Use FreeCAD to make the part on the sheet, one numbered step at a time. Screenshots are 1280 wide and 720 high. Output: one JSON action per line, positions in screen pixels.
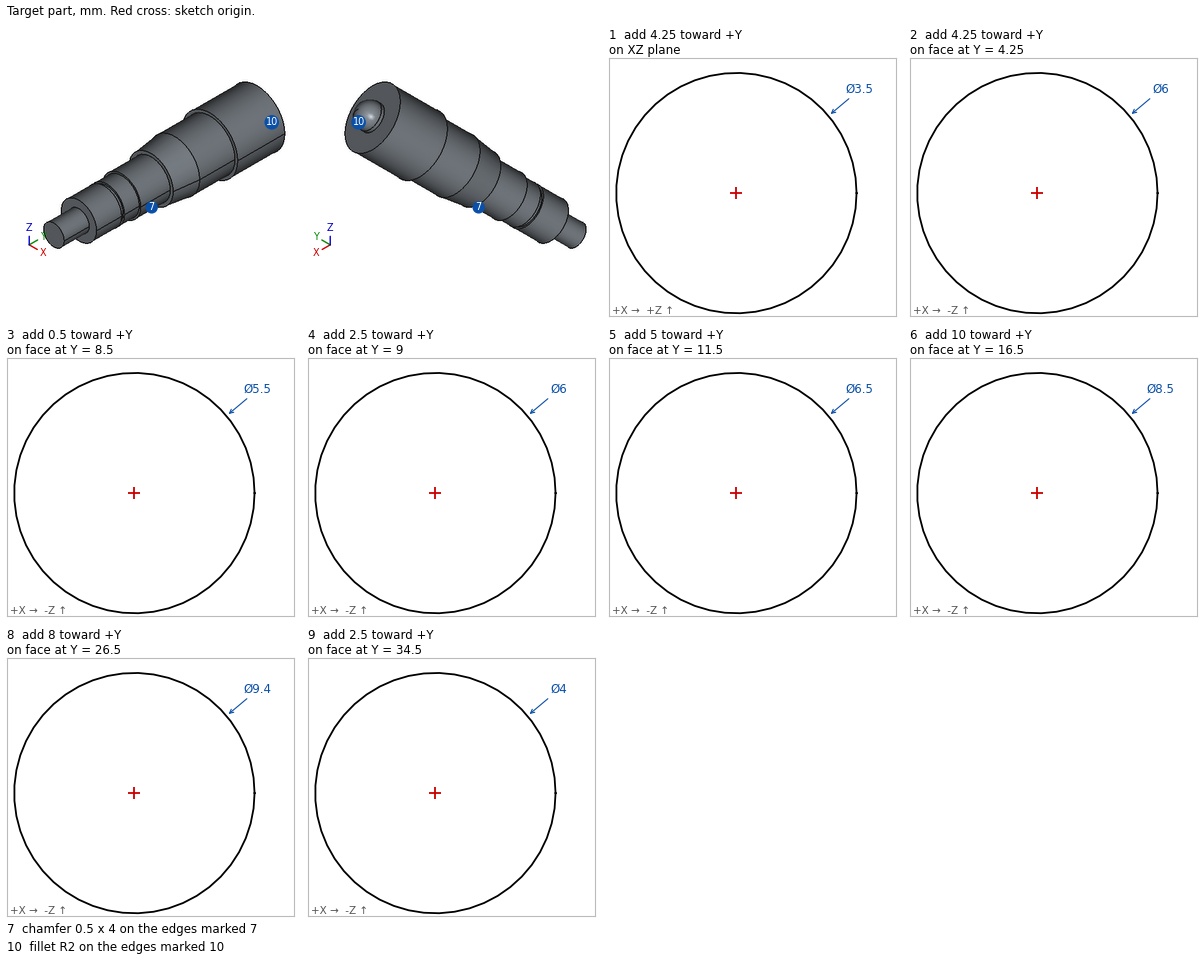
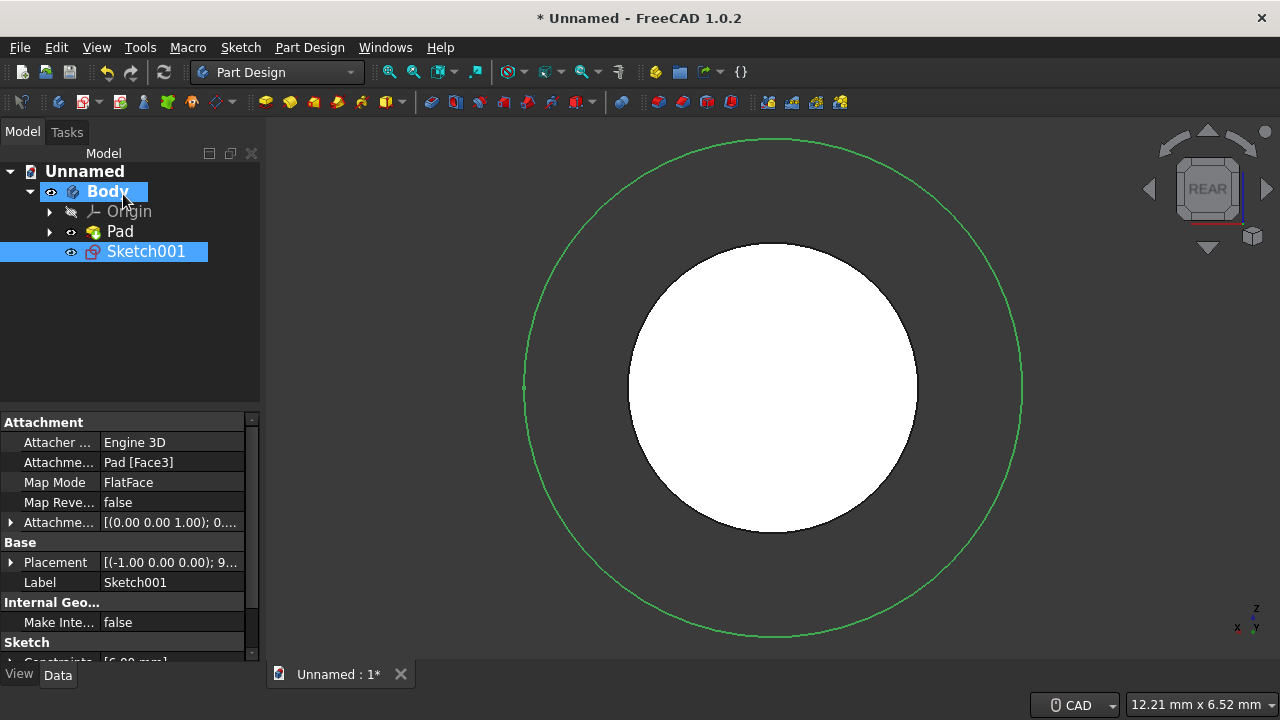
{"action": "left_click", "coordinate": [266, 102]}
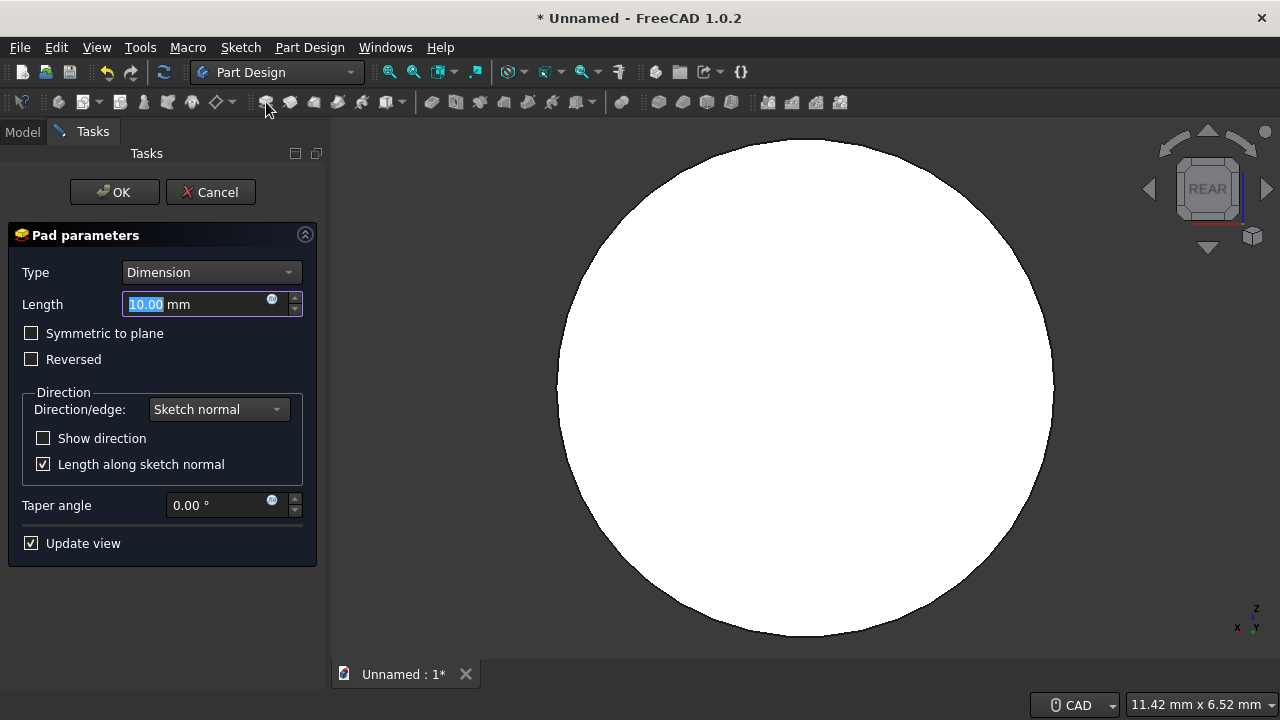
{"action": "type", "text": "4.25"}
{"action": "key", "text": "Tab"}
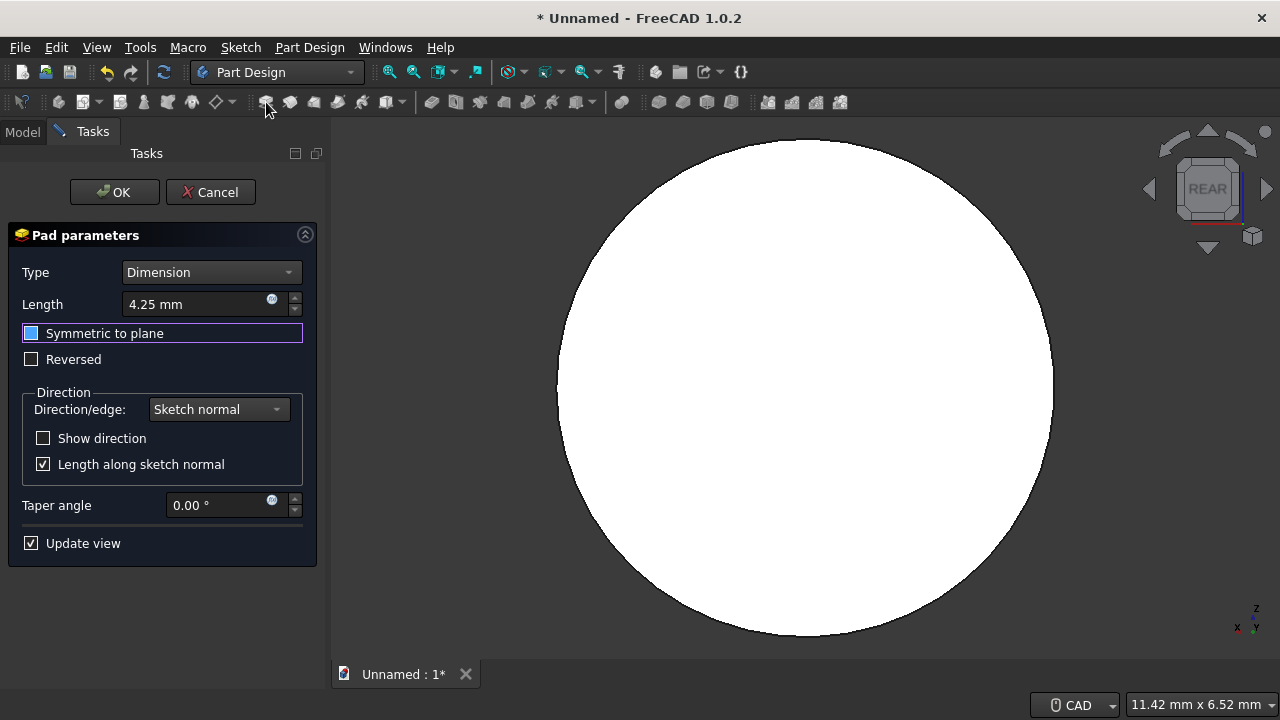
{"action": "left_click", "coordinate": [115, 192]}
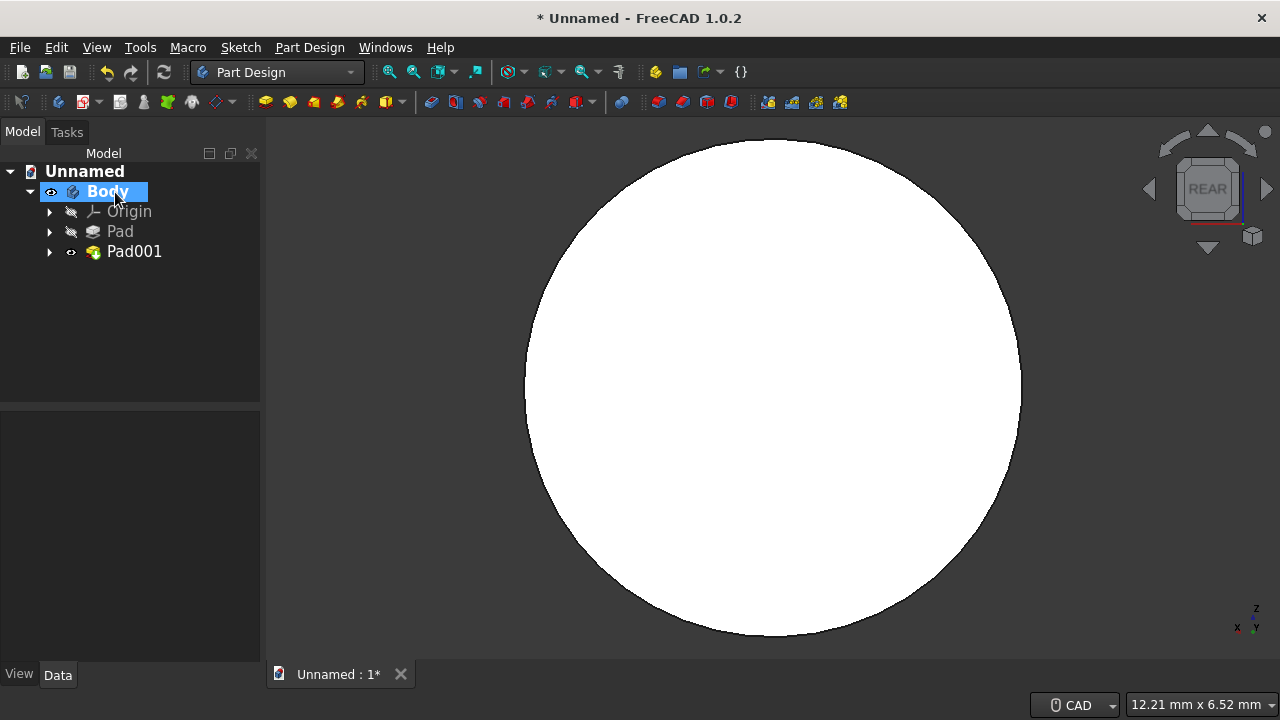
{"action": "left_click", "coordinate": [773, 387]}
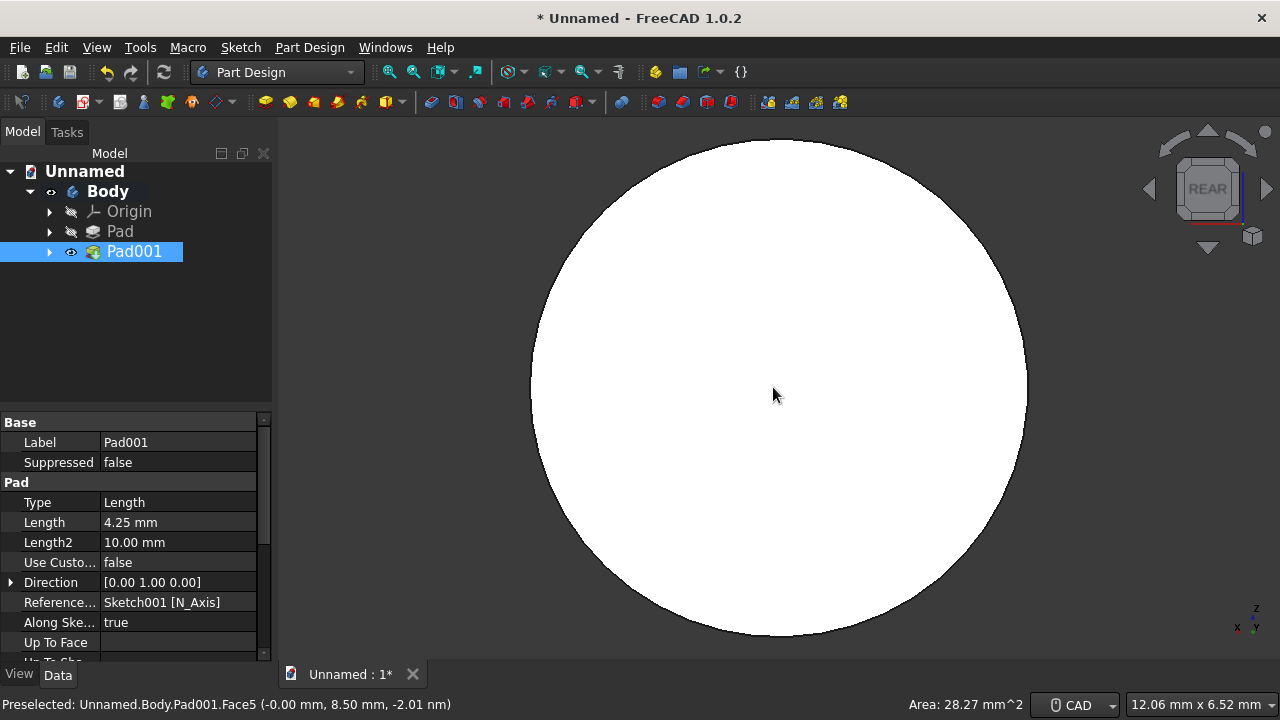
{"action": "left_click", "coordinate": [84, 102]}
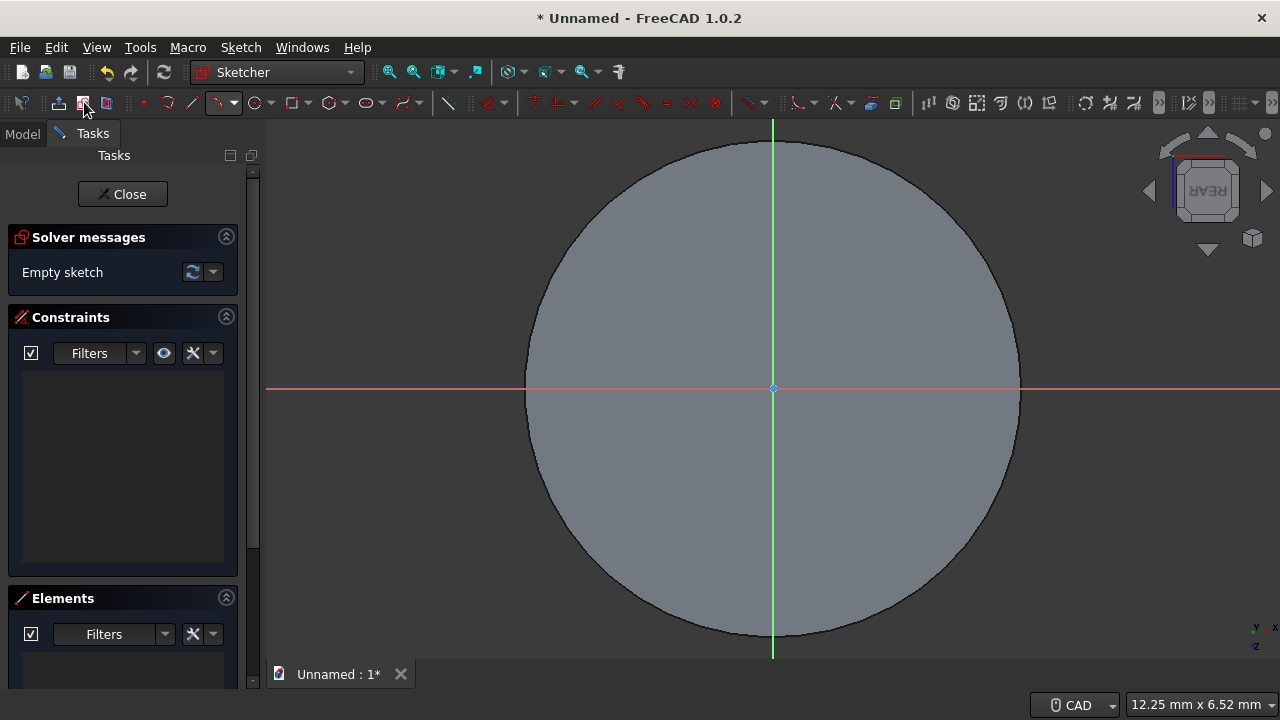
{"action": "scroll", "coordinate": [395, 389], "scroll_direction": "down", "scroll_amount": 1}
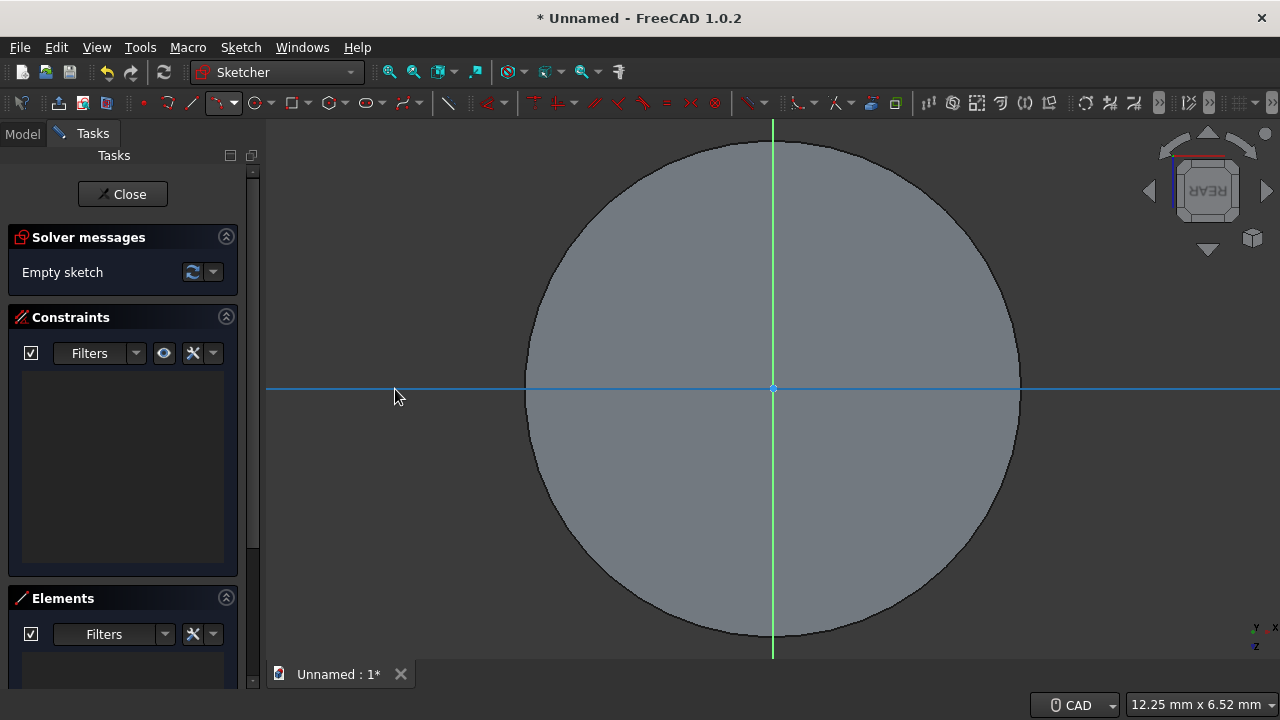
{"action": "left_click", "coordinate": [256, 104]}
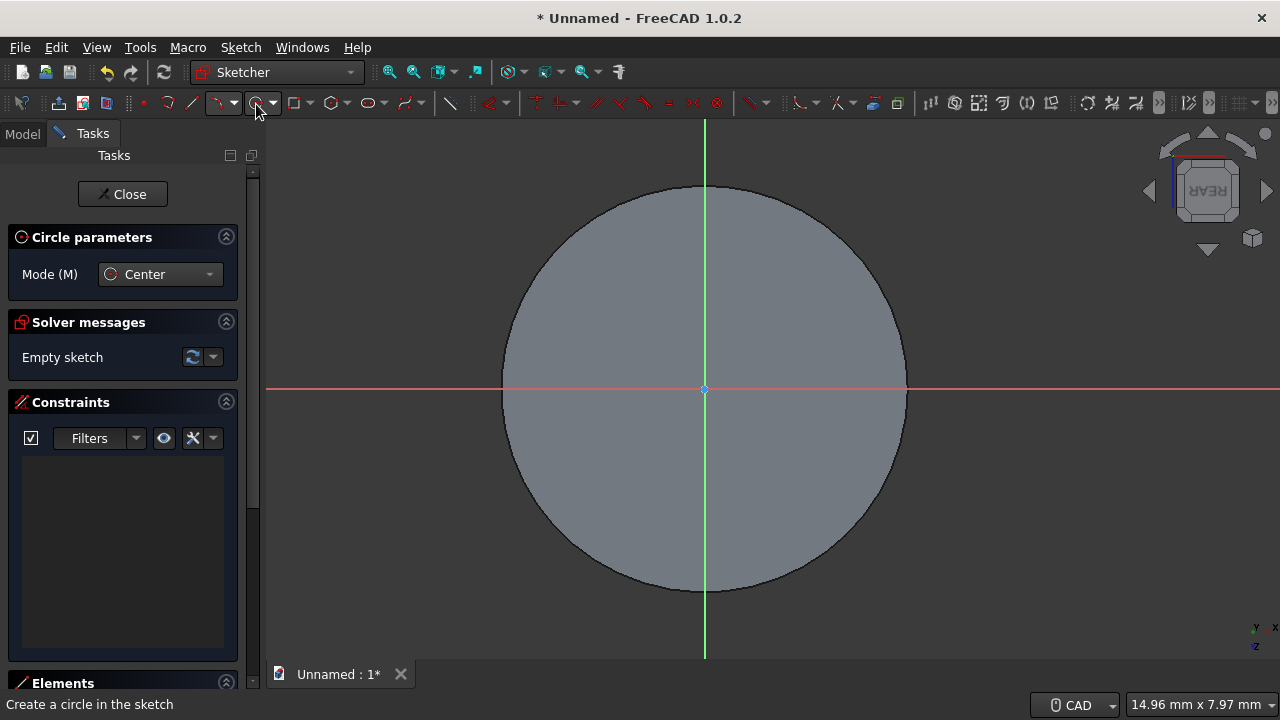
{"action": "left_click", "coordinate": [705, 389]}
{"action": "mouse_move", "coordinate": [836, 257]}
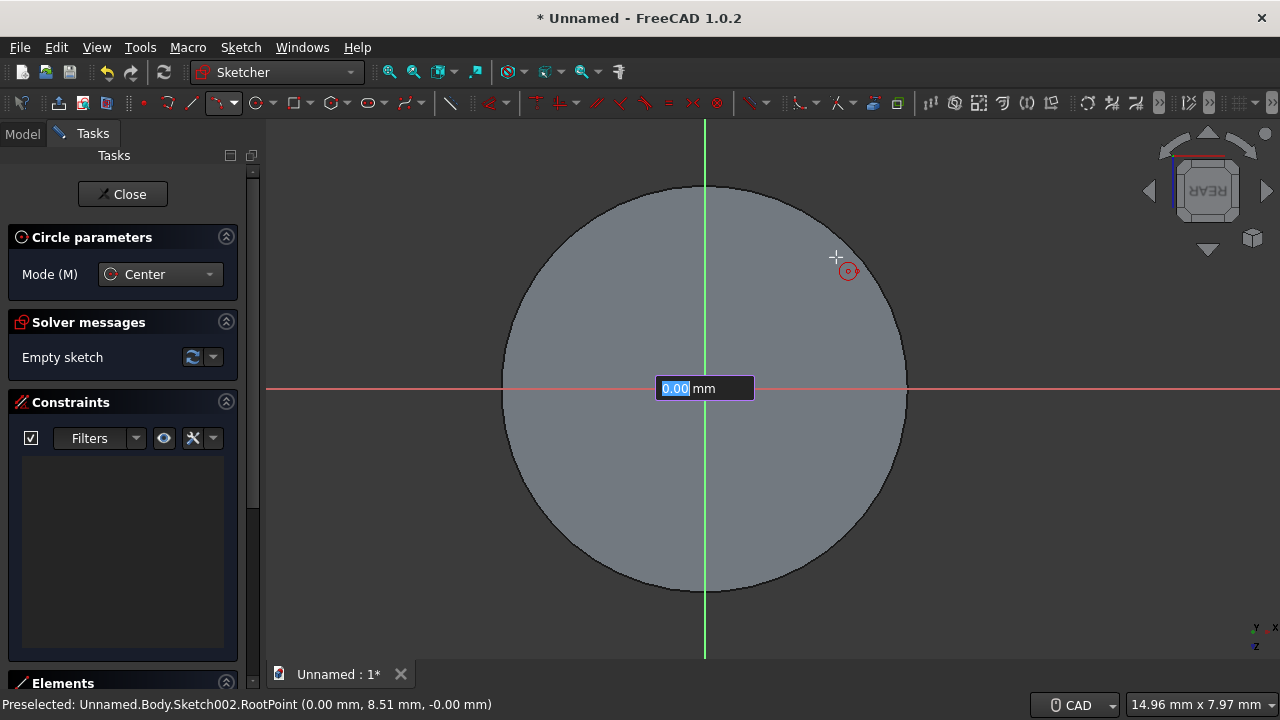
{"action": "type", "text": "5.5"}
{"action": "key", "text": "Return"}
{"action": "key", "text": "Escape"}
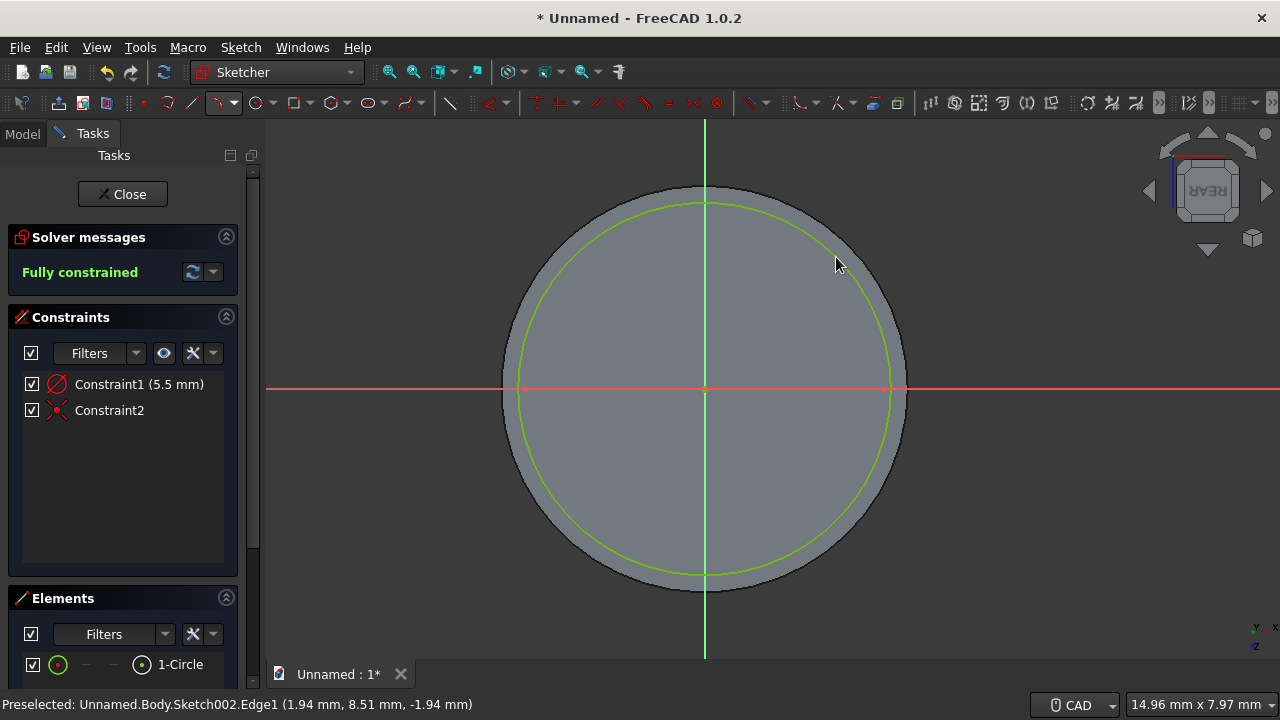
{"action": "left_click", "coordinate": [123, 194]}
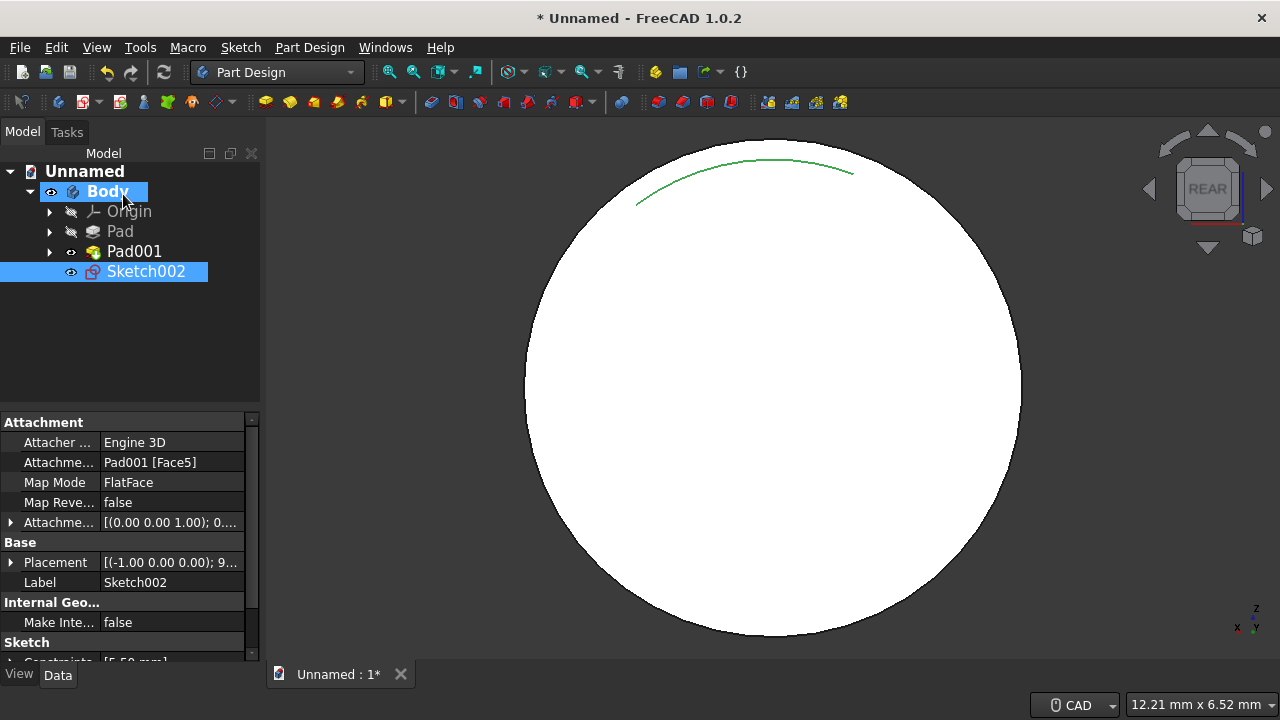
{"action": "left_click", "coordinate": [266, 102]}